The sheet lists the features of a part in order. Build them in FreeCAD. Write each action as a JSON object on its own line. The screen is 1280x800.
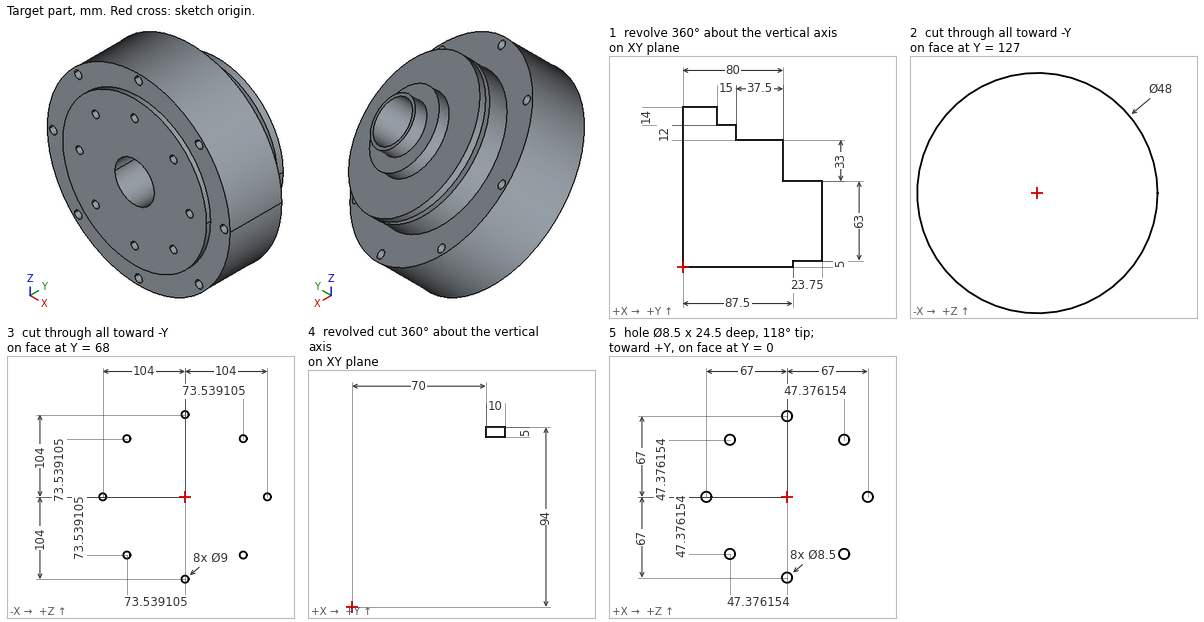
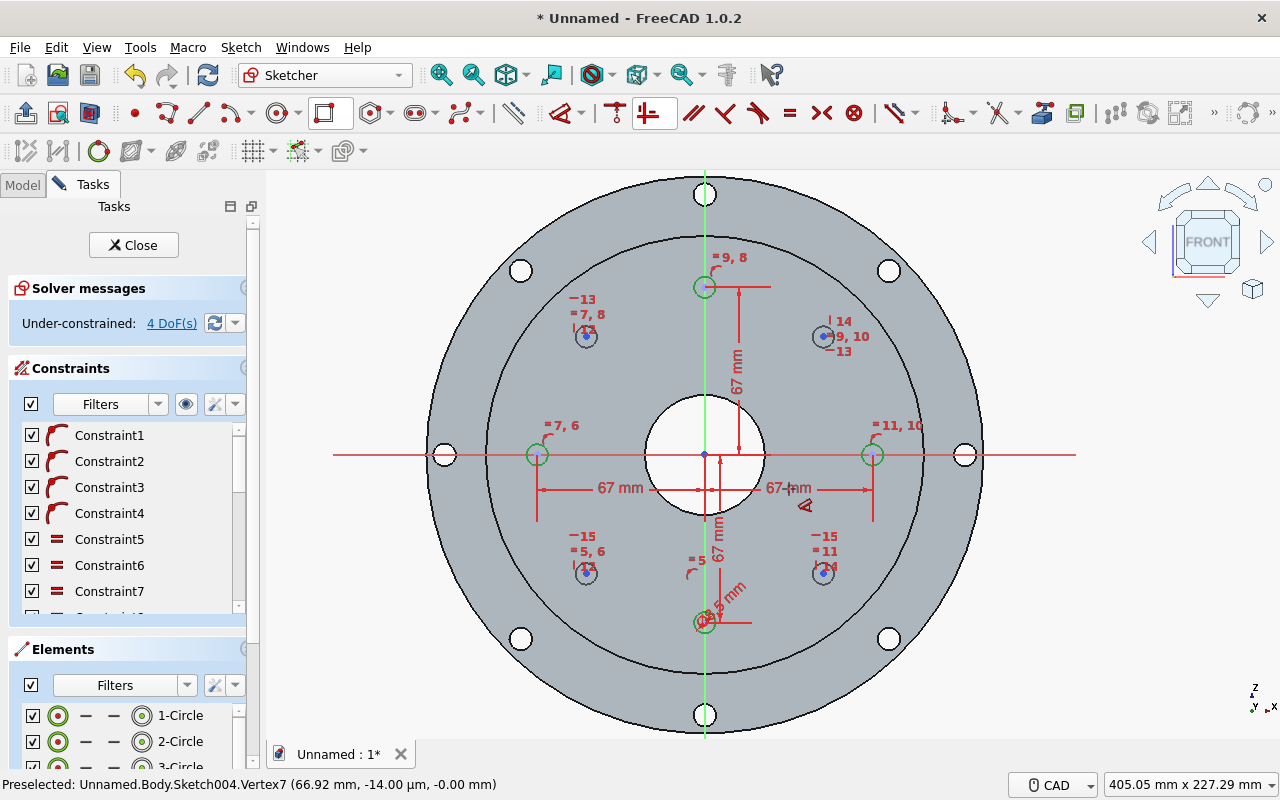
{"action": "left_click", "coordinate": [586, 574]}
{"action": "left_click", "coordinate": [646, 608]}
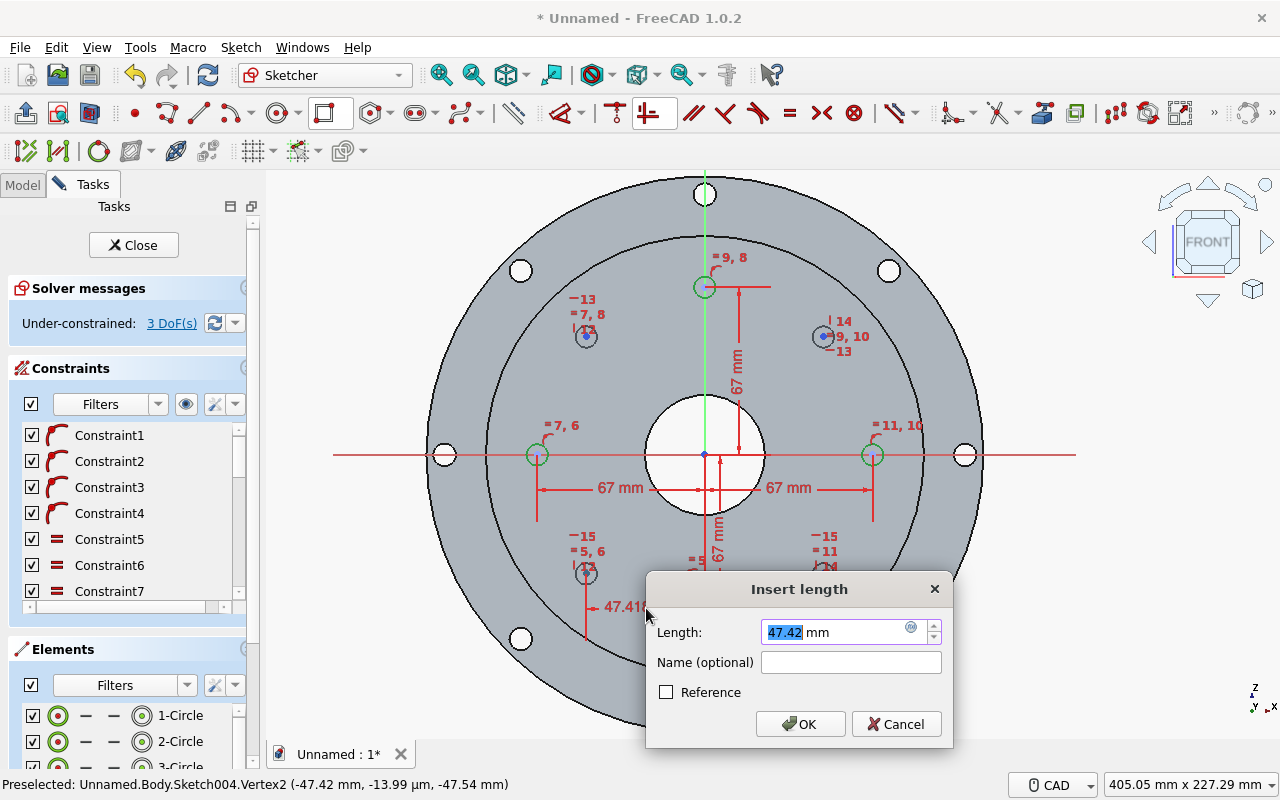
{"action": "type", "text": "47.376154"}
{"action": "key", "text": "Return"}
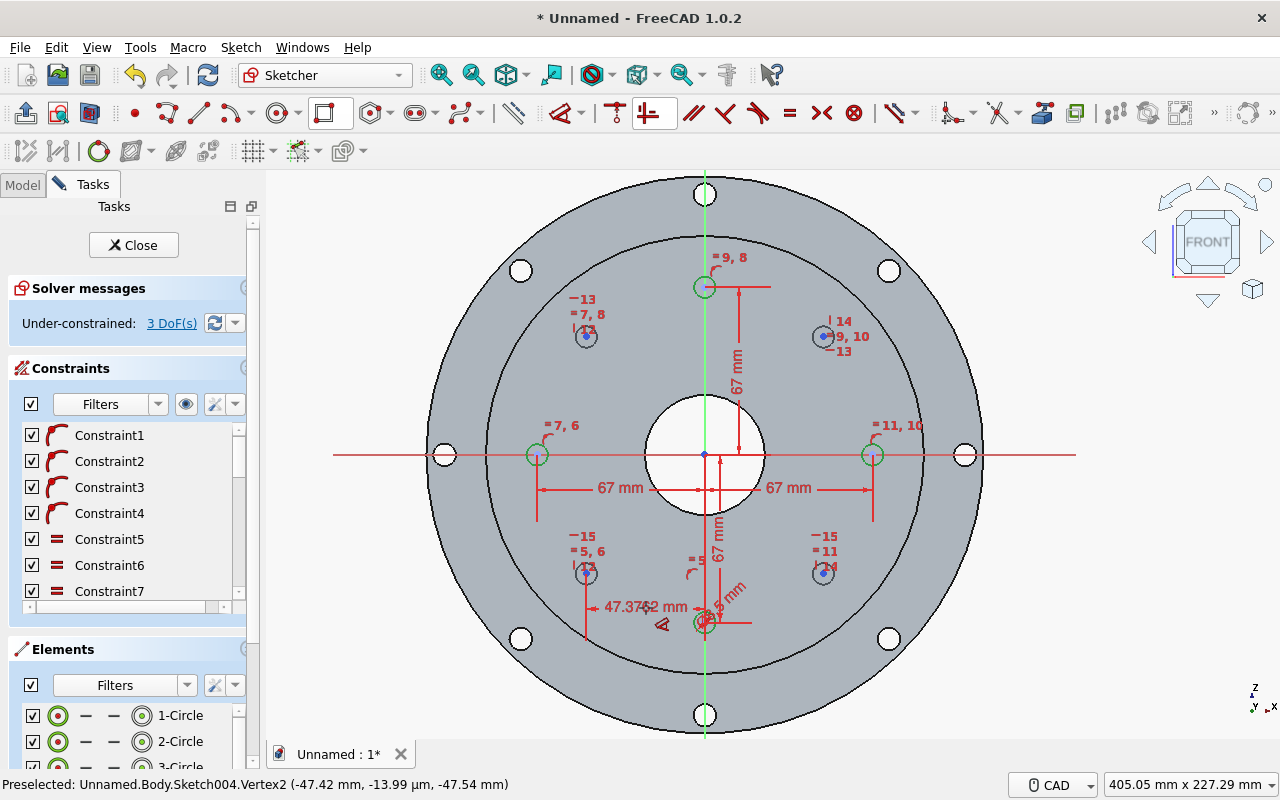
{"action": "left_click", "coordinate": [586, 574]}
{"action": "left_click", "coordinate": [552, 514]}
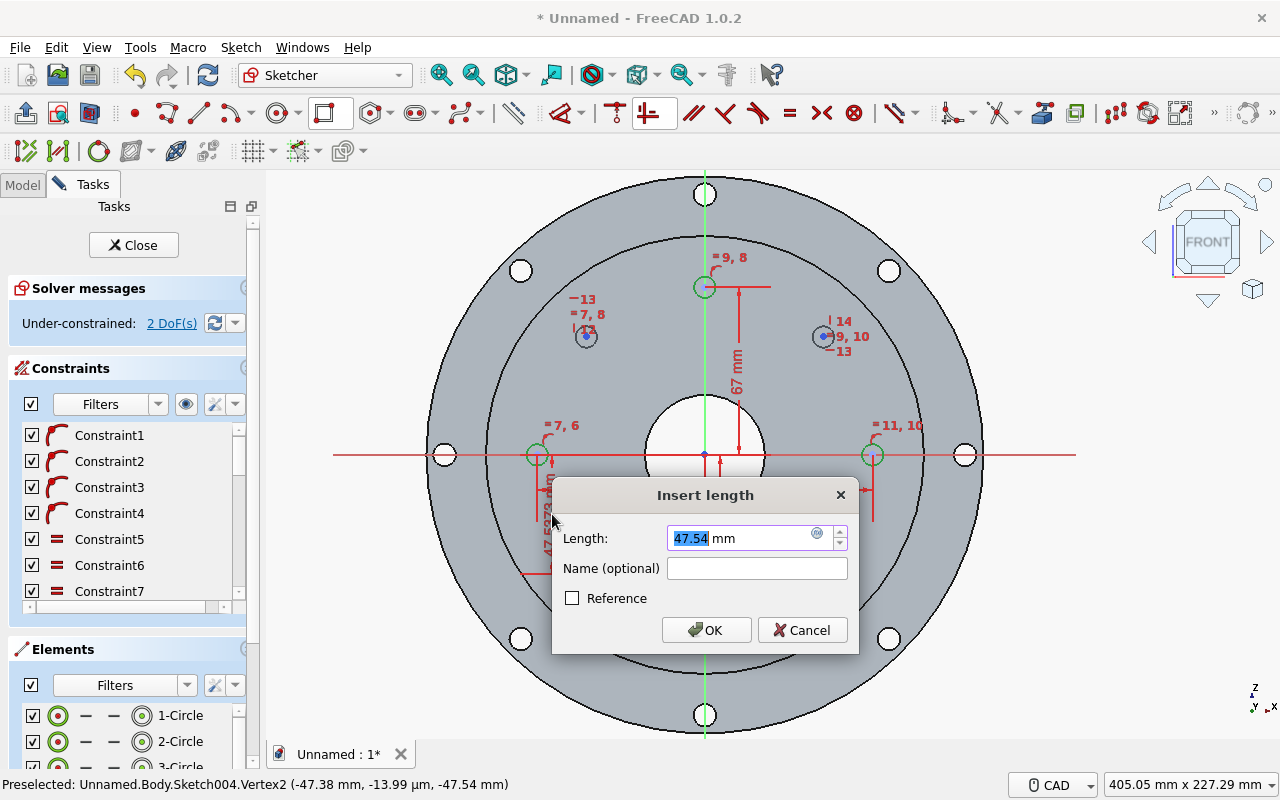
{"action": "type", "text": "47.376154"}
{"action": "key", "text": "Return"}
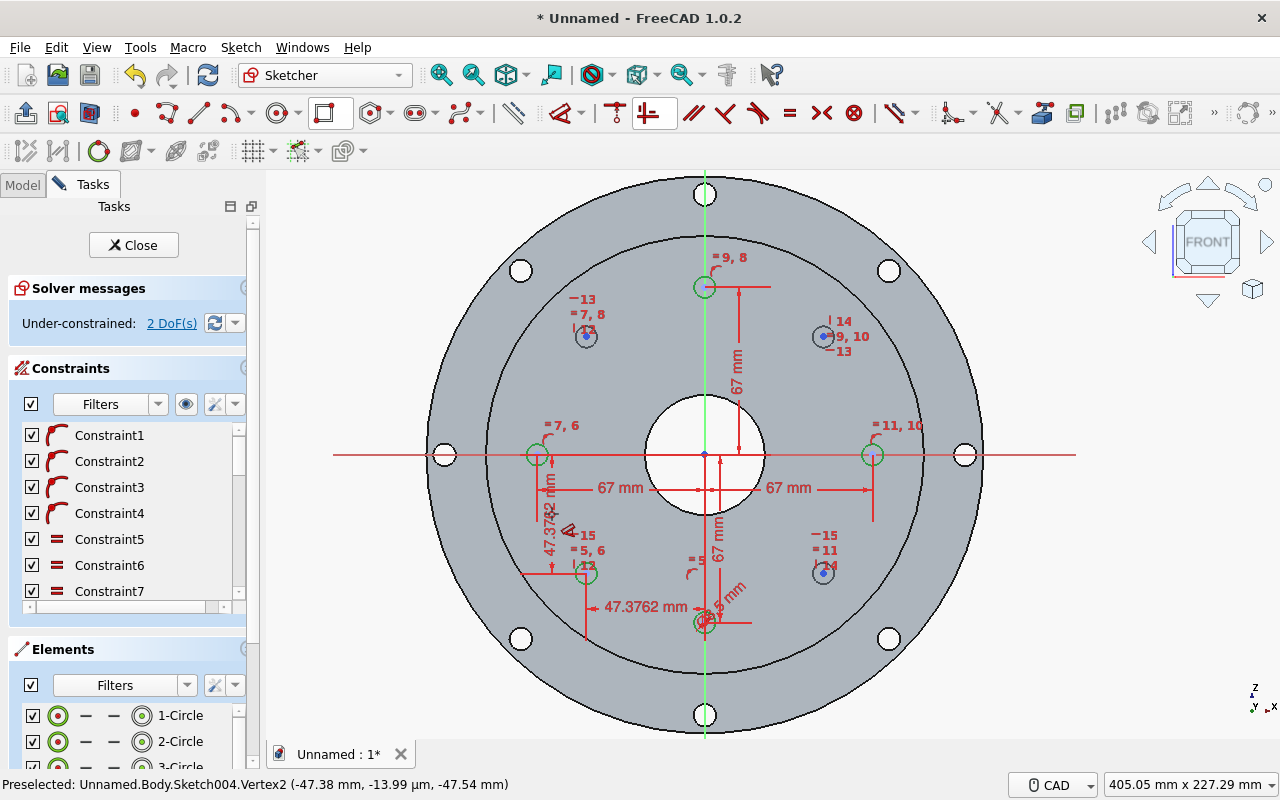
{"action": "left_click", "coordinate": [586, 337]}
{"action": "left_click", "coordinate": [552, 396]}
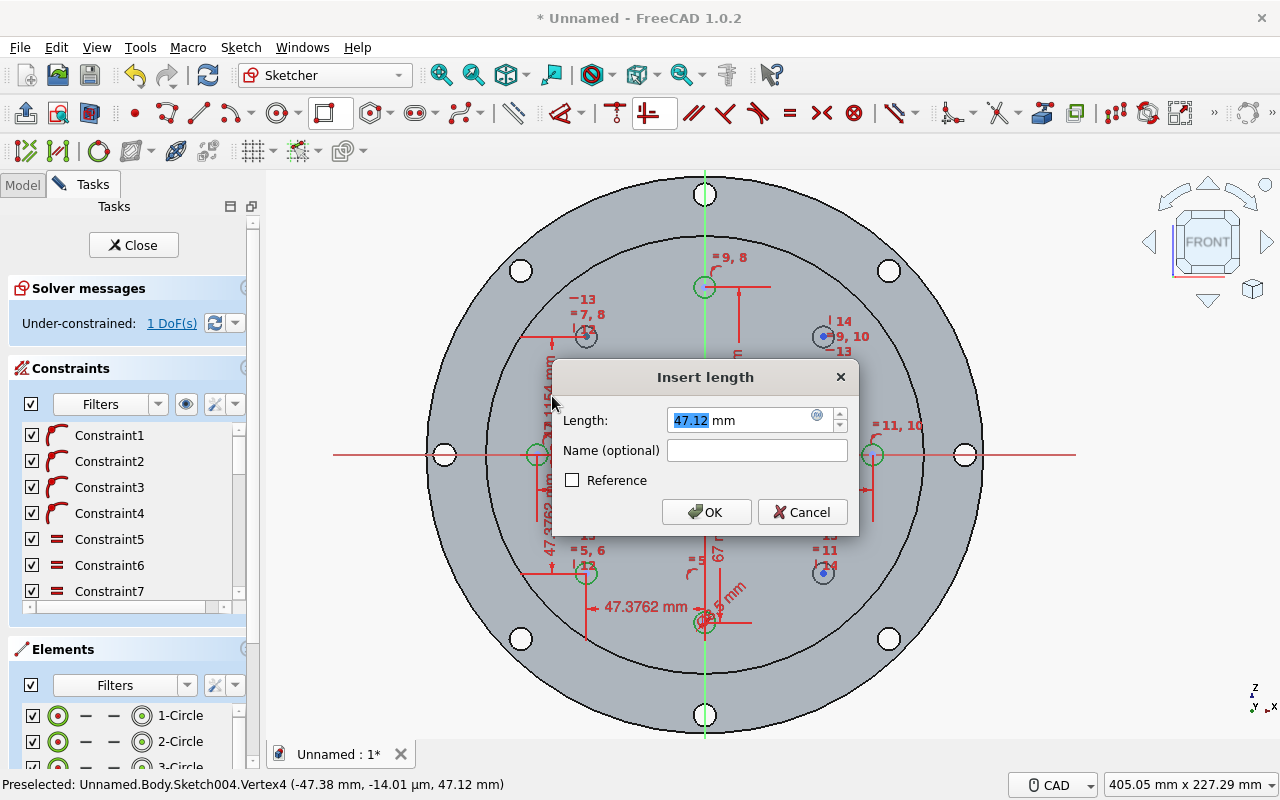
{"action": "type", "text": "47.376154"}
{"action": "key", "text": "Return"}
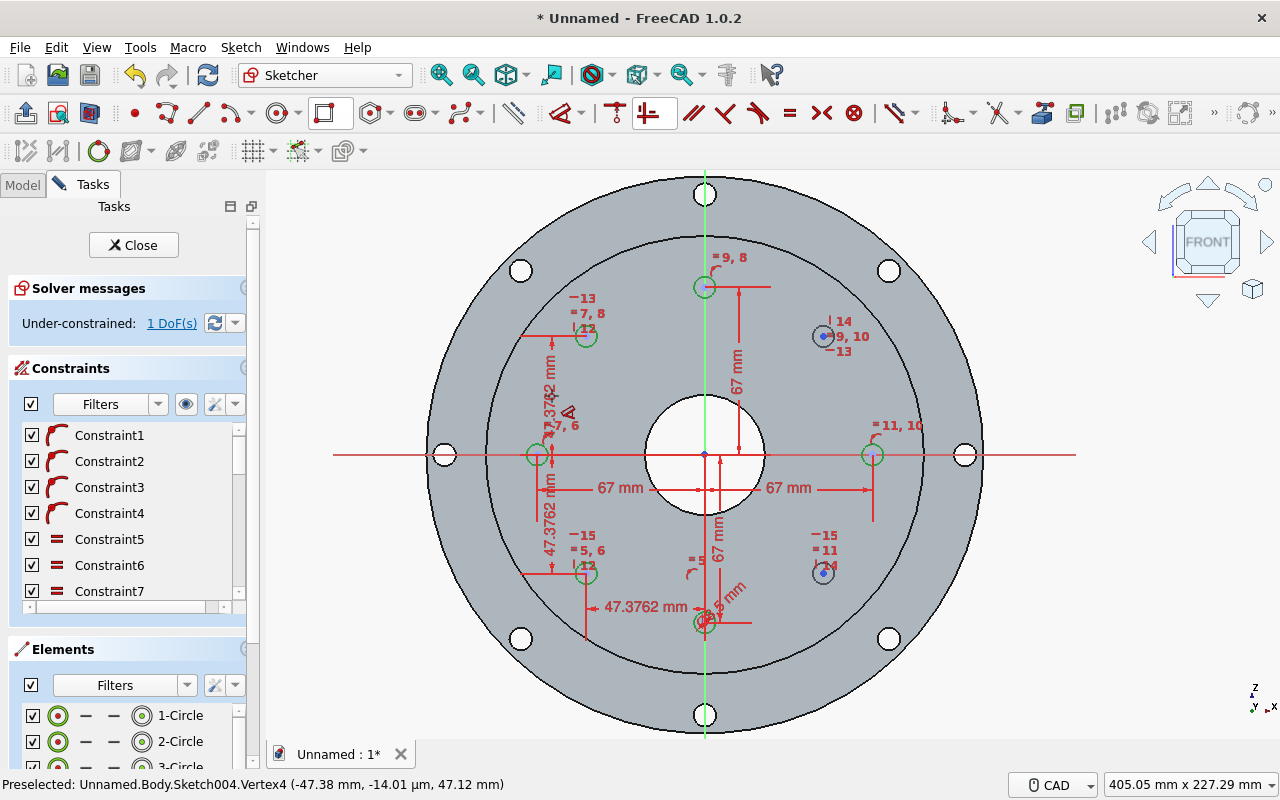
{"action": "left_click", "coordinate": [823, 336]}
{"action": "left_click", "coordinate": [764, 302]}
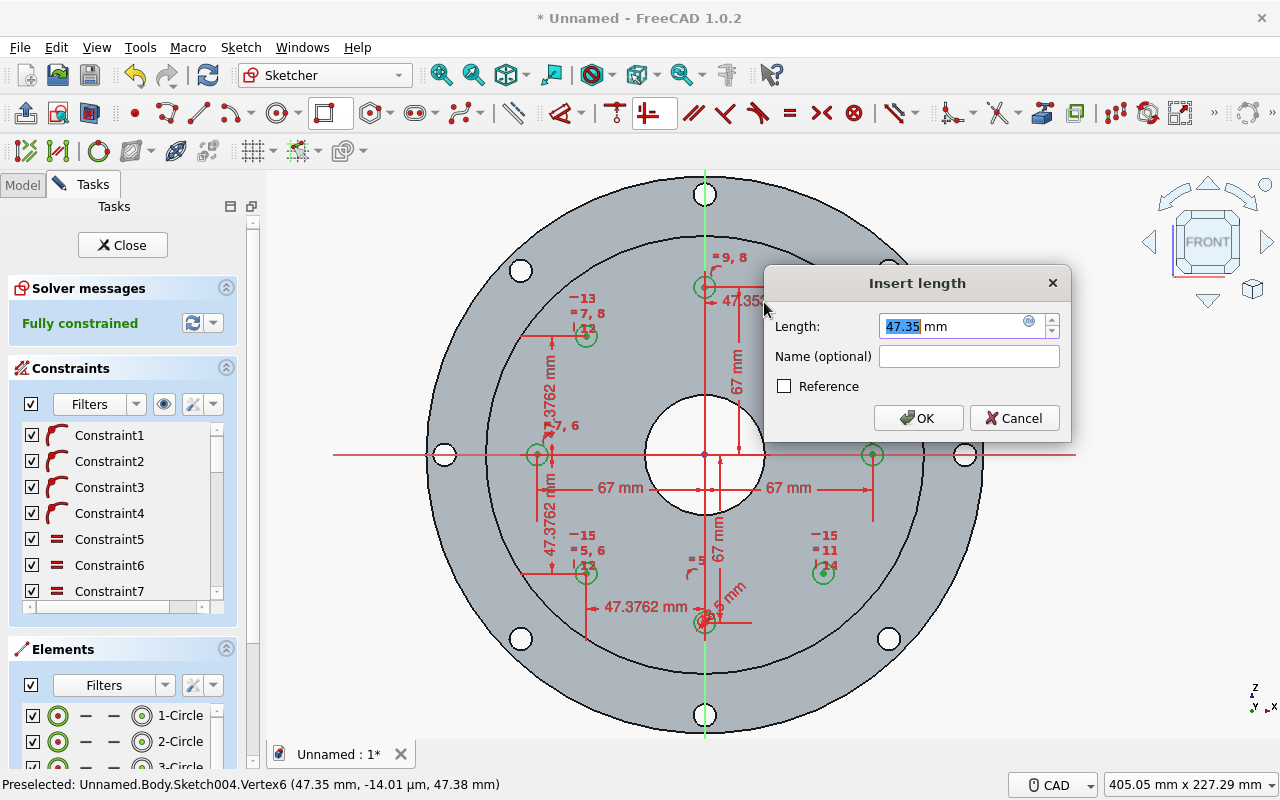
{"action": "type", "text": "47.376154"}
{"action": "key", "text": "Return"}
{"action": "key", "text": "Escape"}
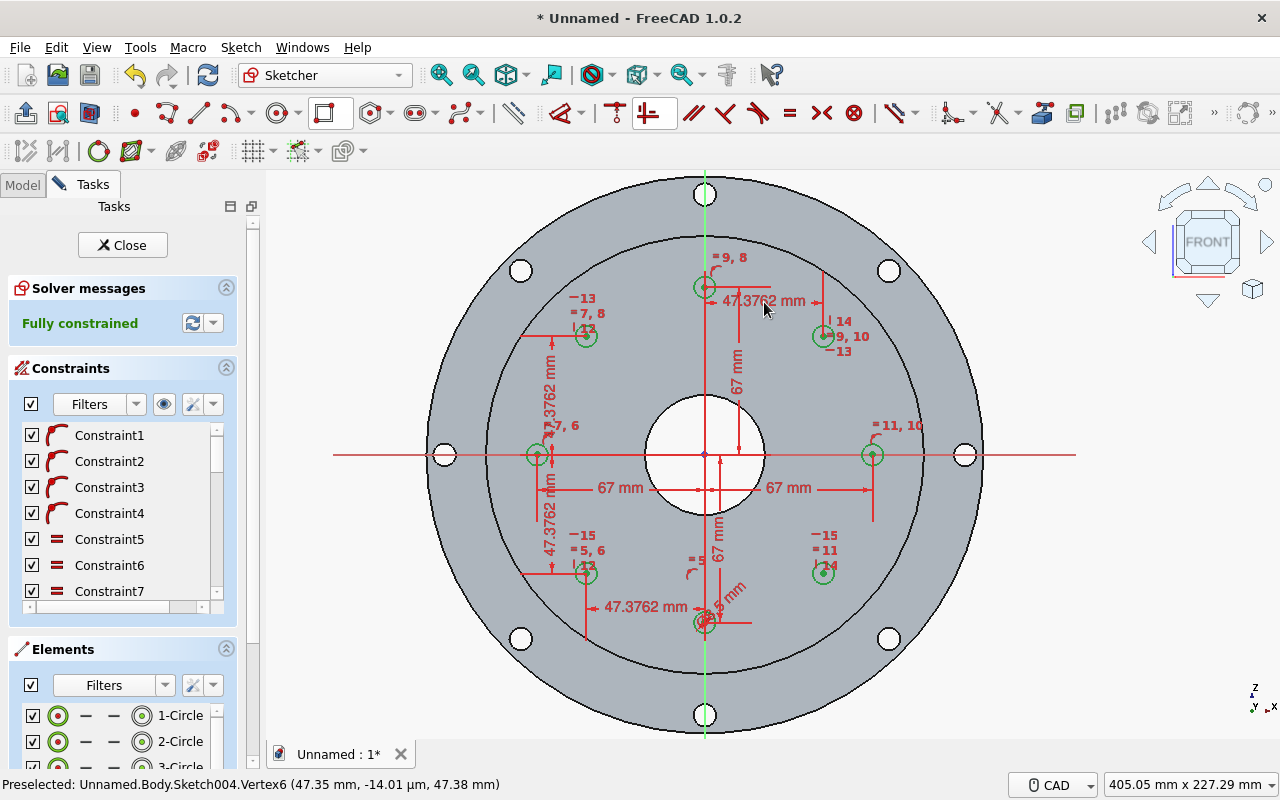
{"action": "left_click", "coordinate": [123, 245]}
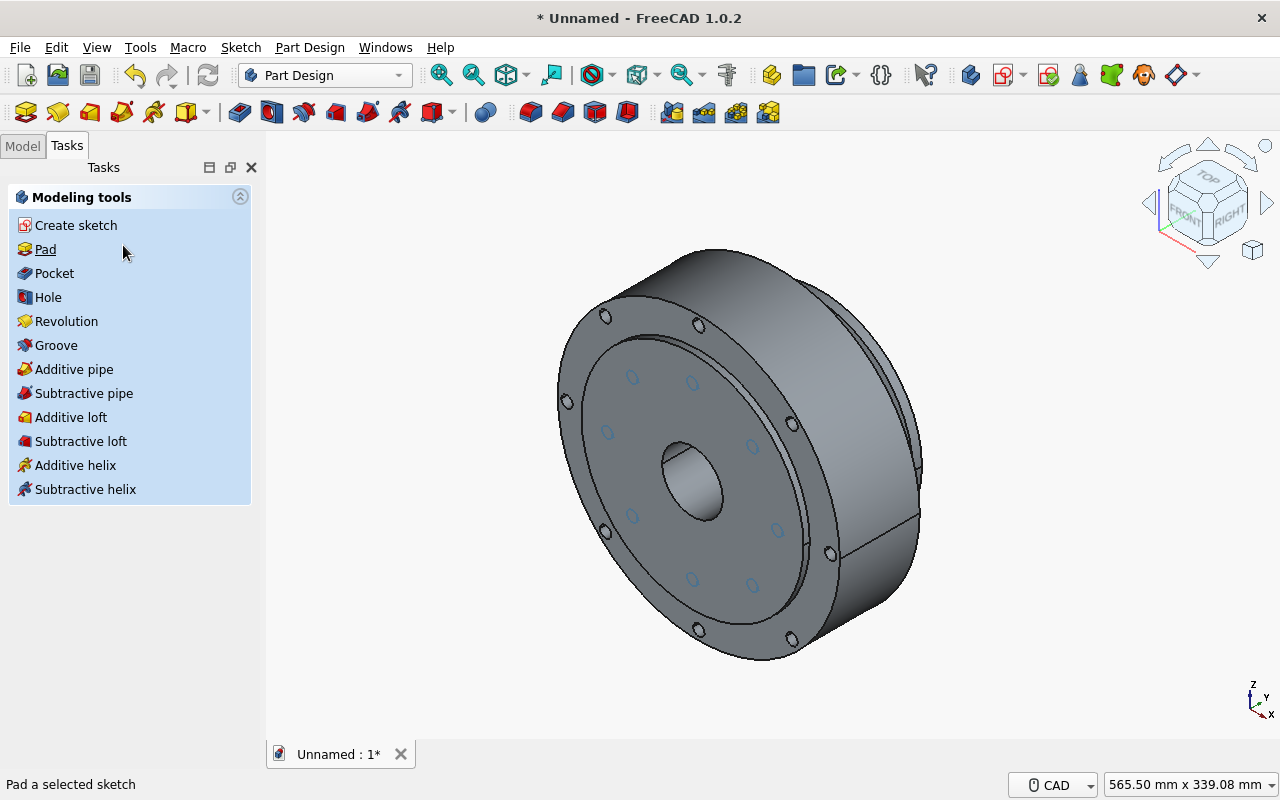
{"action": "left_click", "coordinate": [272, 112]}